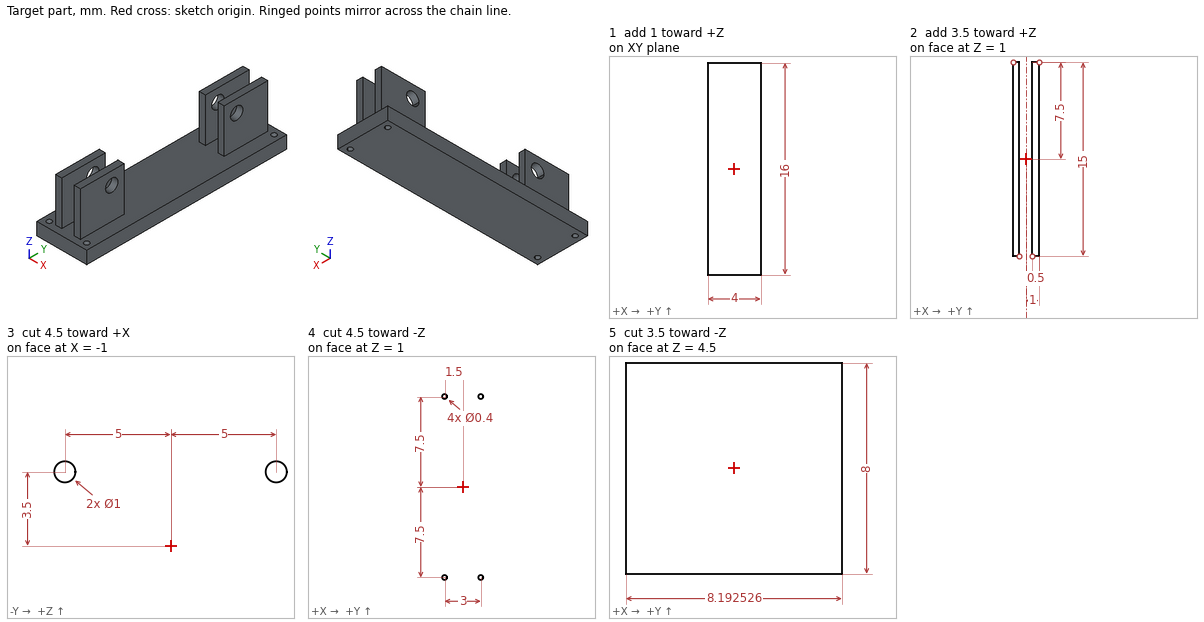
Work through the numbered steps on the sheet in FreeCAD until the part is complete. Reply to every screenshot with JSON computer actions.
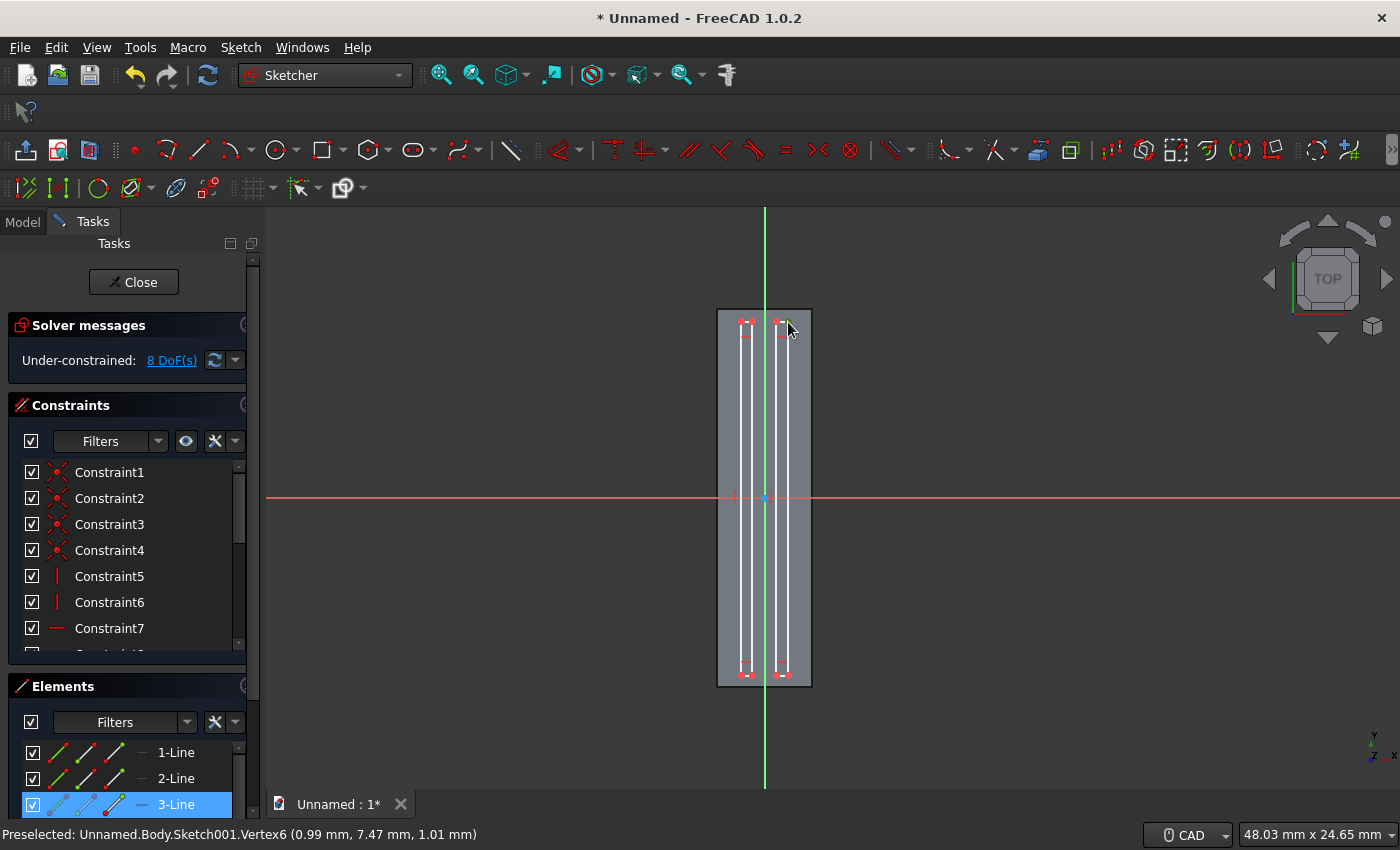
{"action": "left_click", "coordinate": [741, 322]}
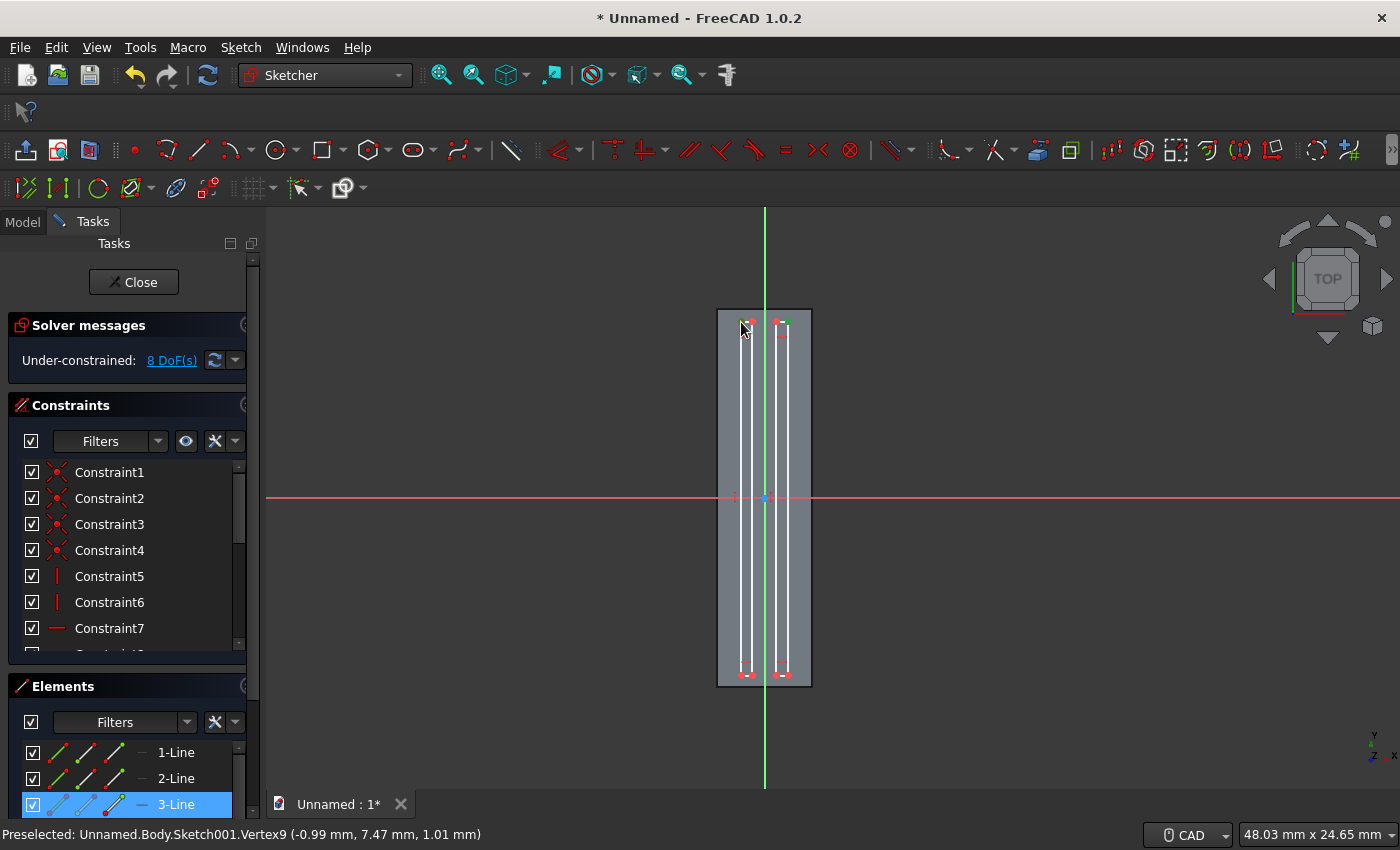
{"action": "left_click", "coordinate": [765, 723]}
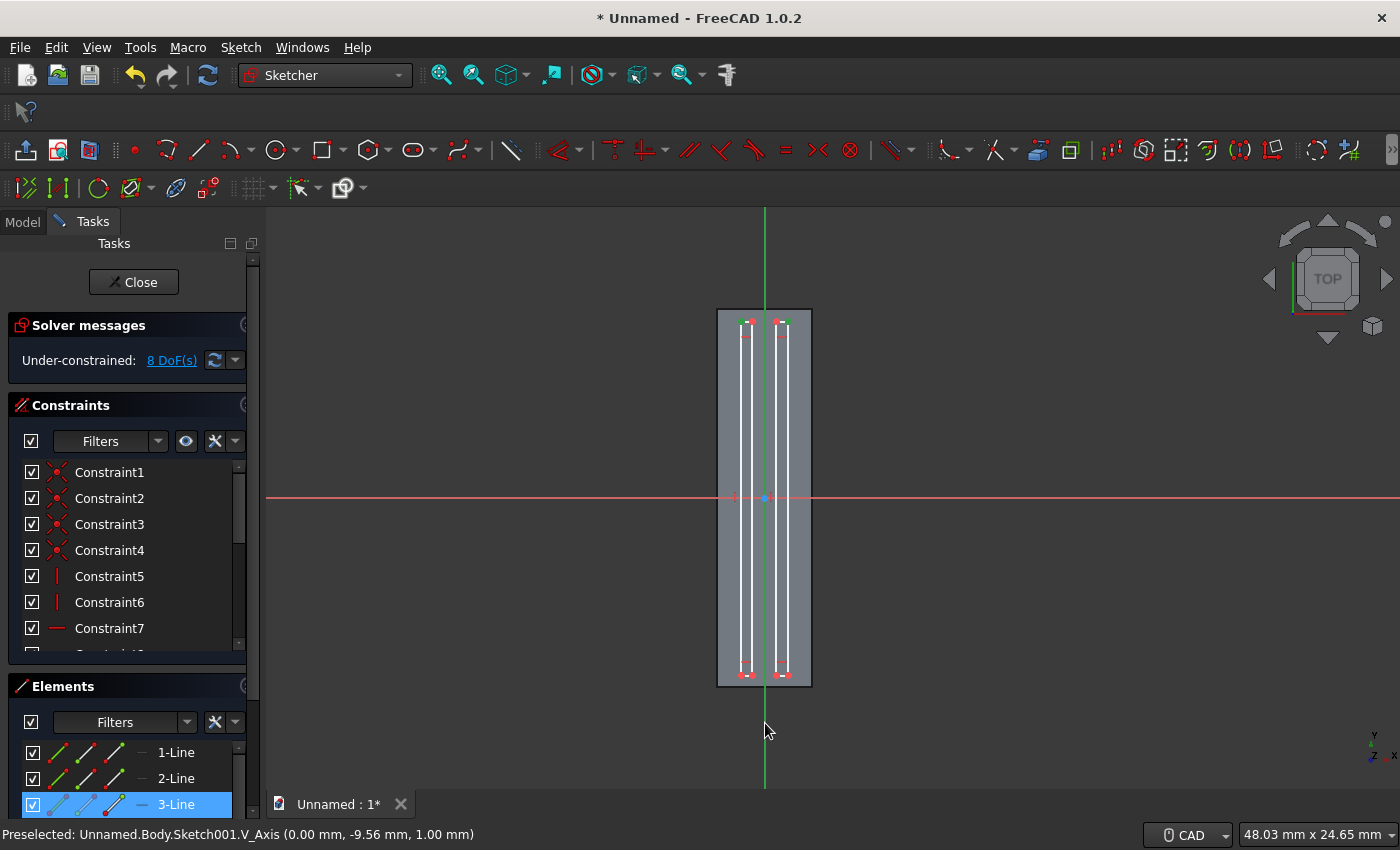
{"action": "left_click", "coordinate": [818, 150]}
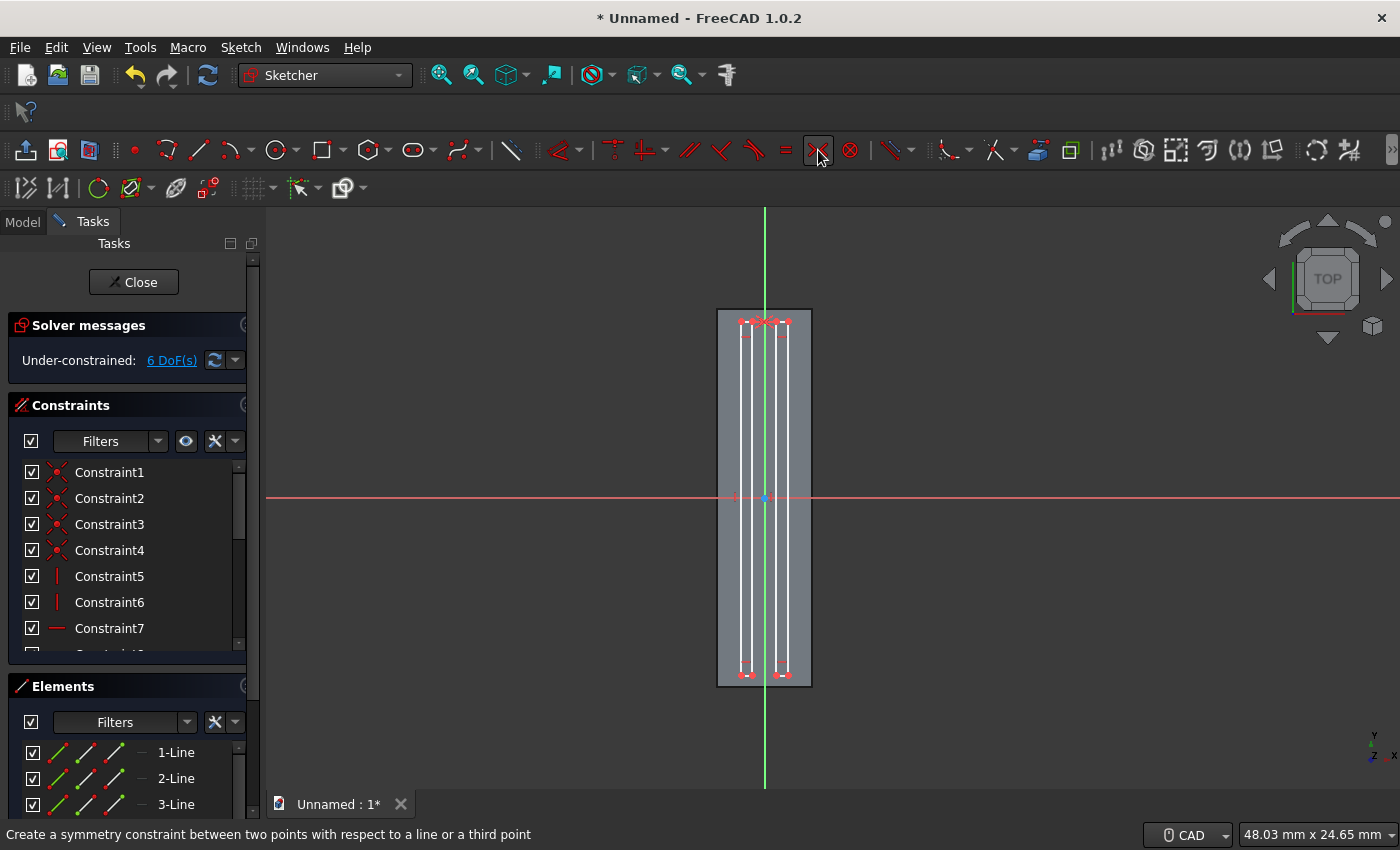
{"action": "left_click", "coordinate": [776, 676]}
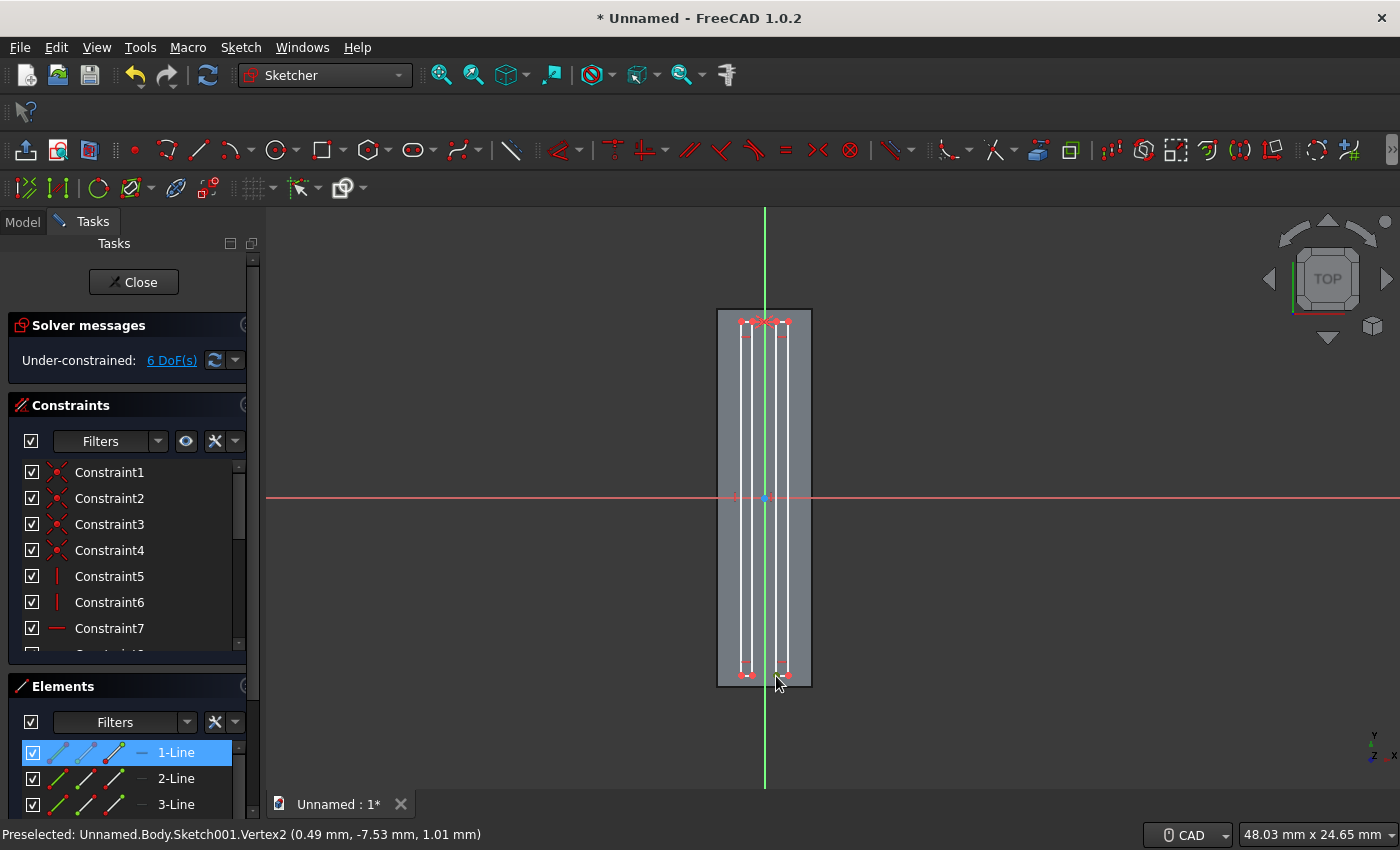
{"action": "left_click", "coordinate": [752, 676]}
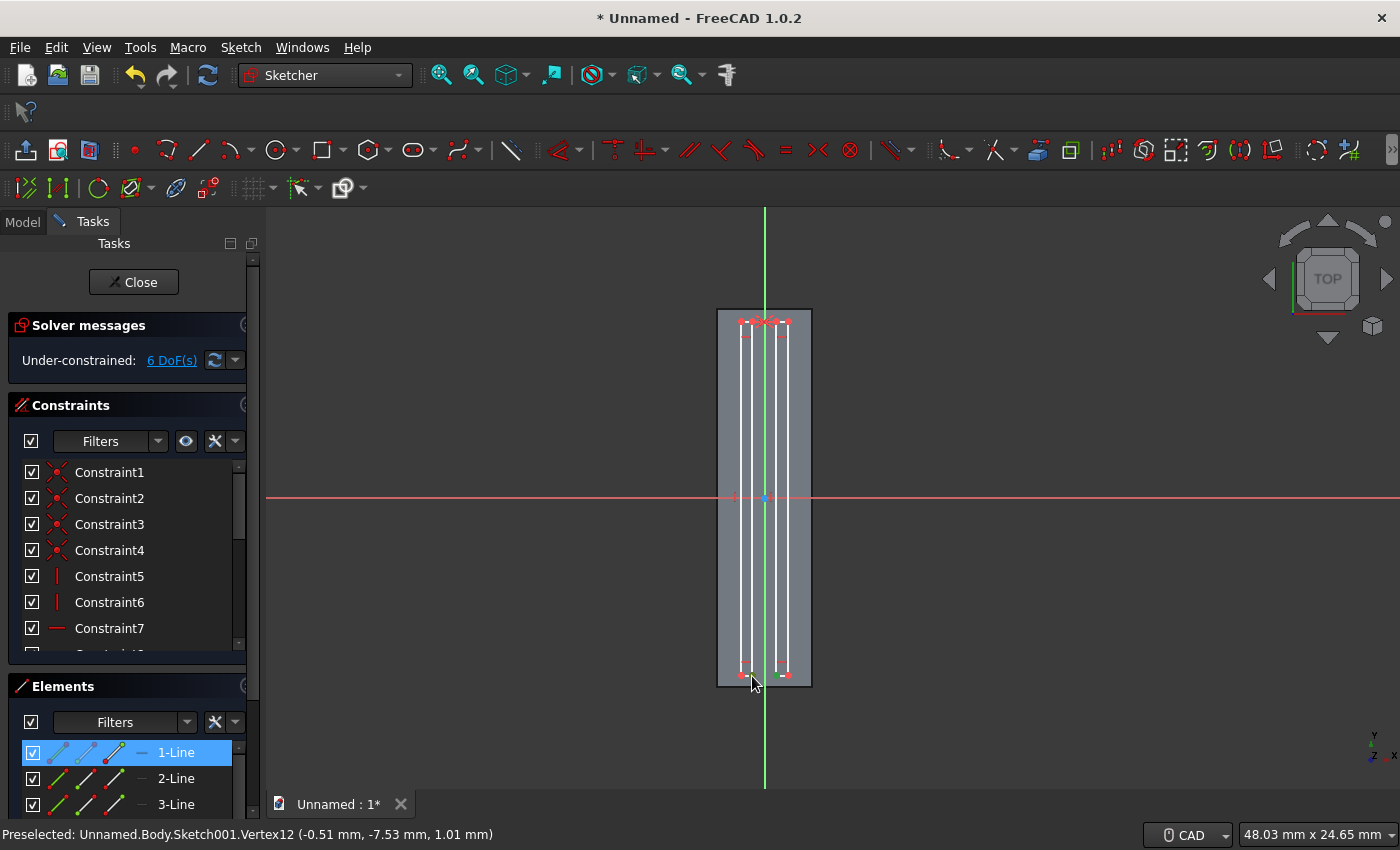
{"action": "left_click", "coordinate": [765, 723]}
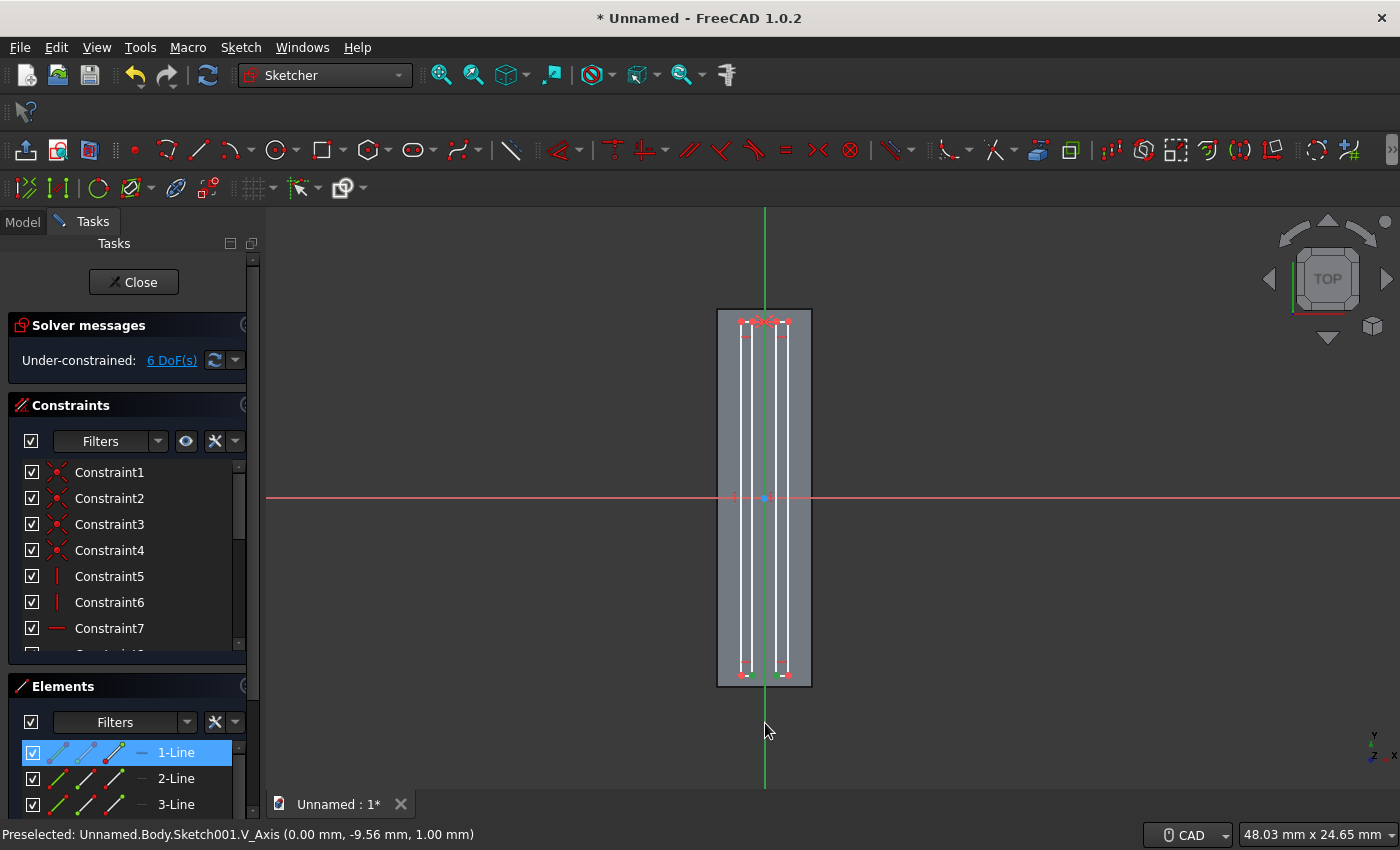
{"action": "key", "text": "s"}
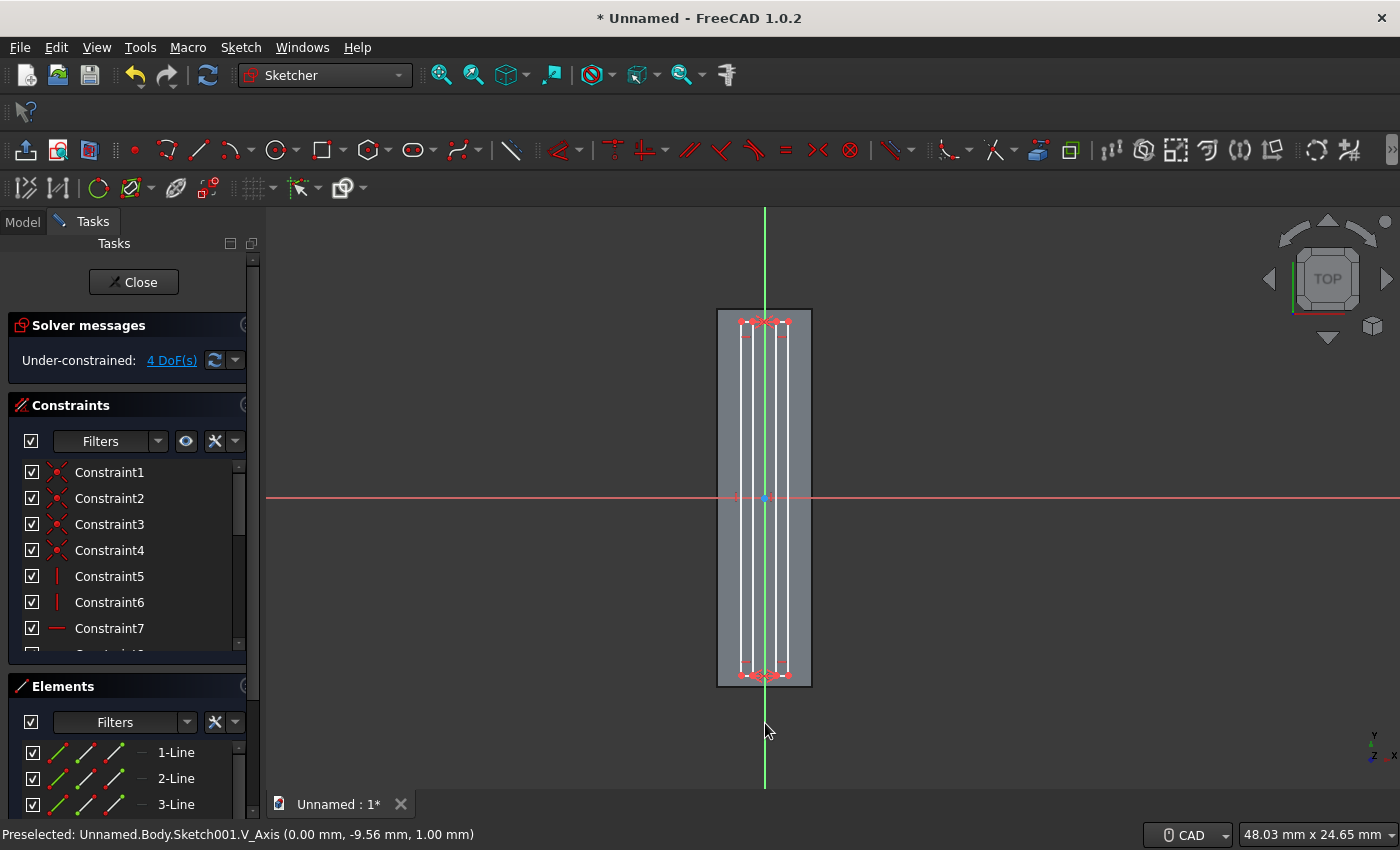
{"action": "left_click", "coordinate": [558, 150]}